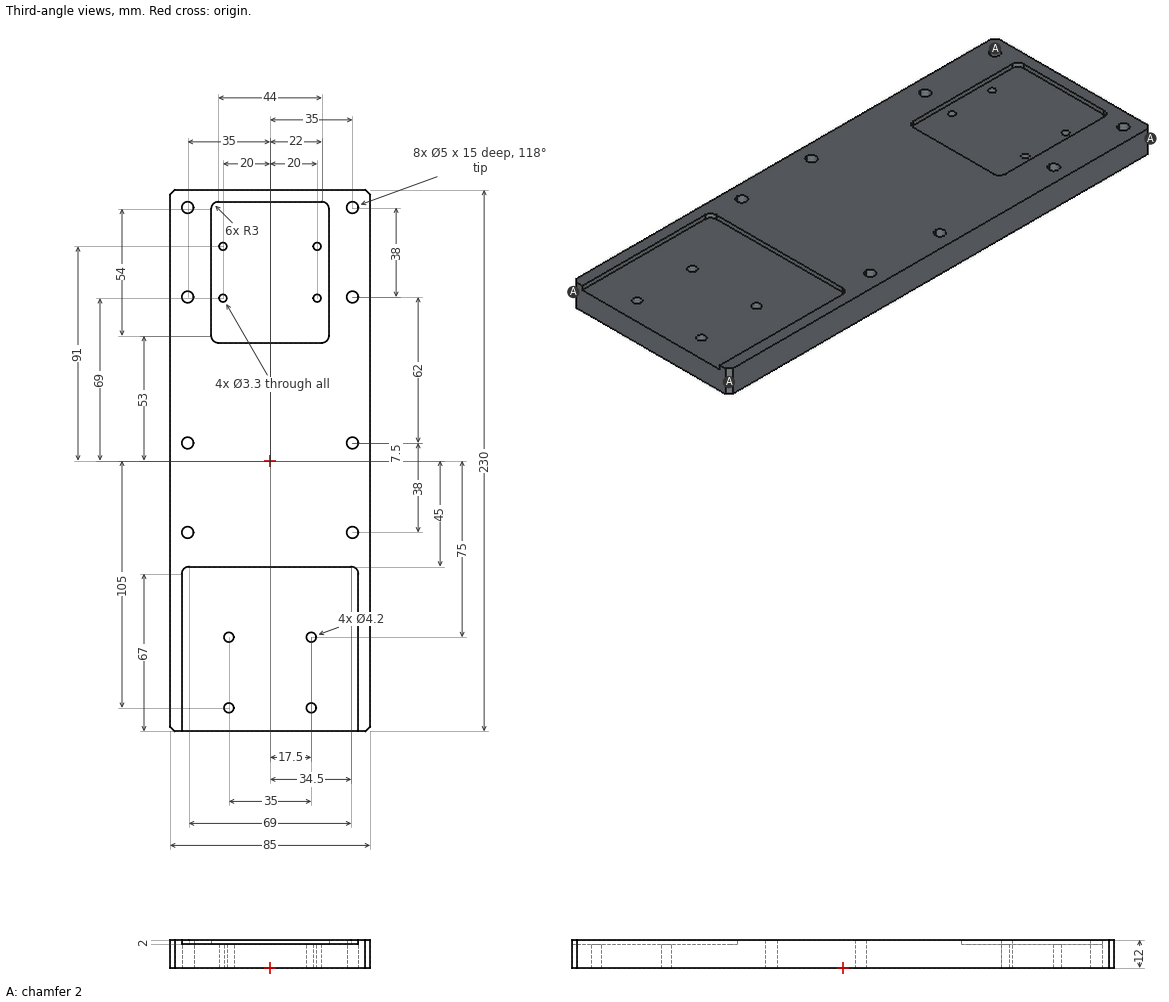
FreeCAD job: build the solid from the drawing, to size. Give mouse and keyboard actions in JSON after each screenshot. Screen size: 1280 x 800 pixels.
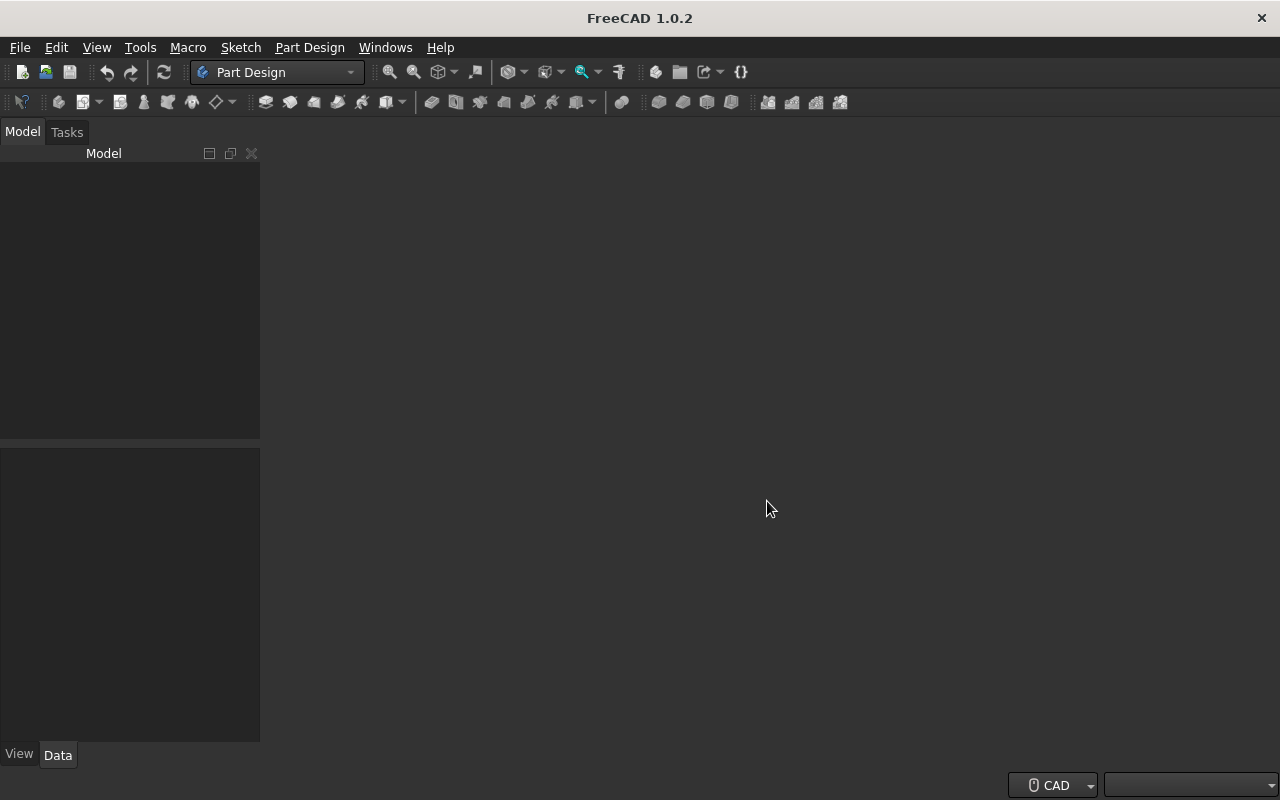
{"action": "key", "text": "ctrl+n"}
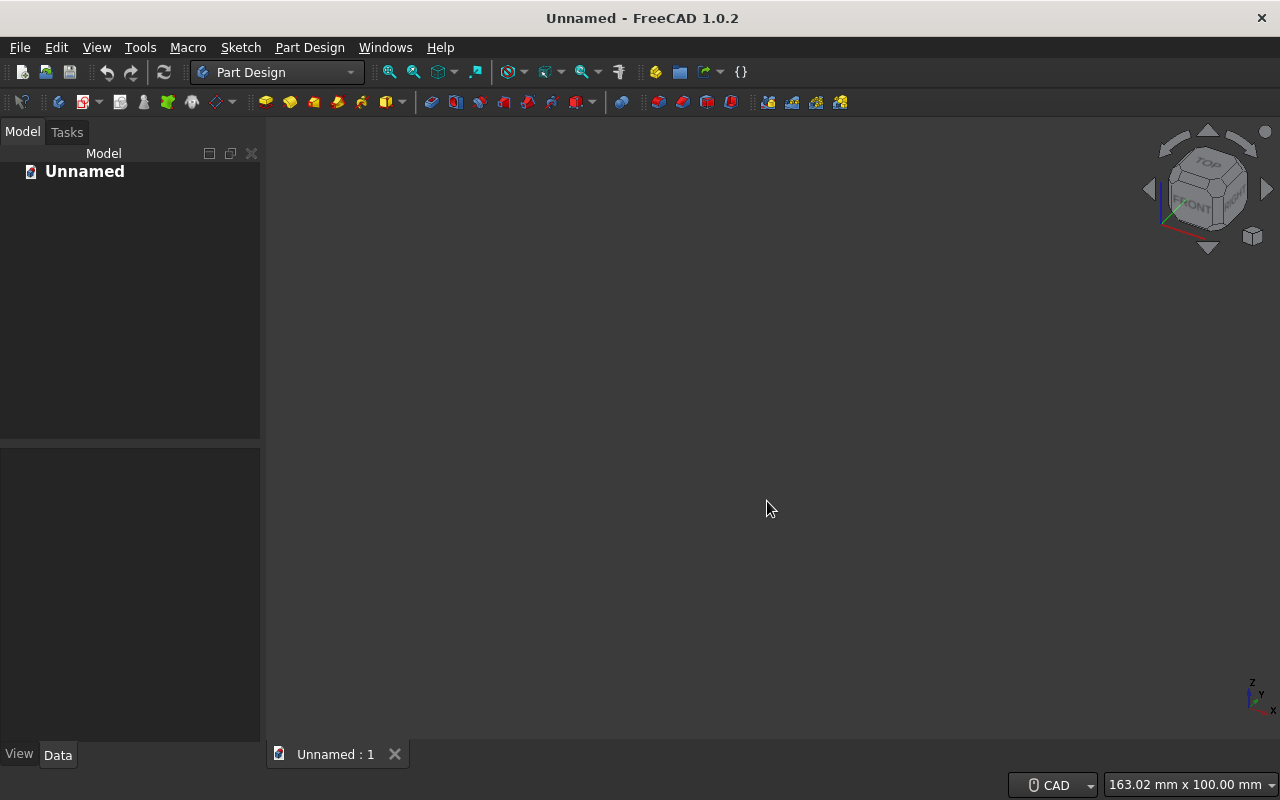
{"action": "left_click", "coordinate": [84, 102]}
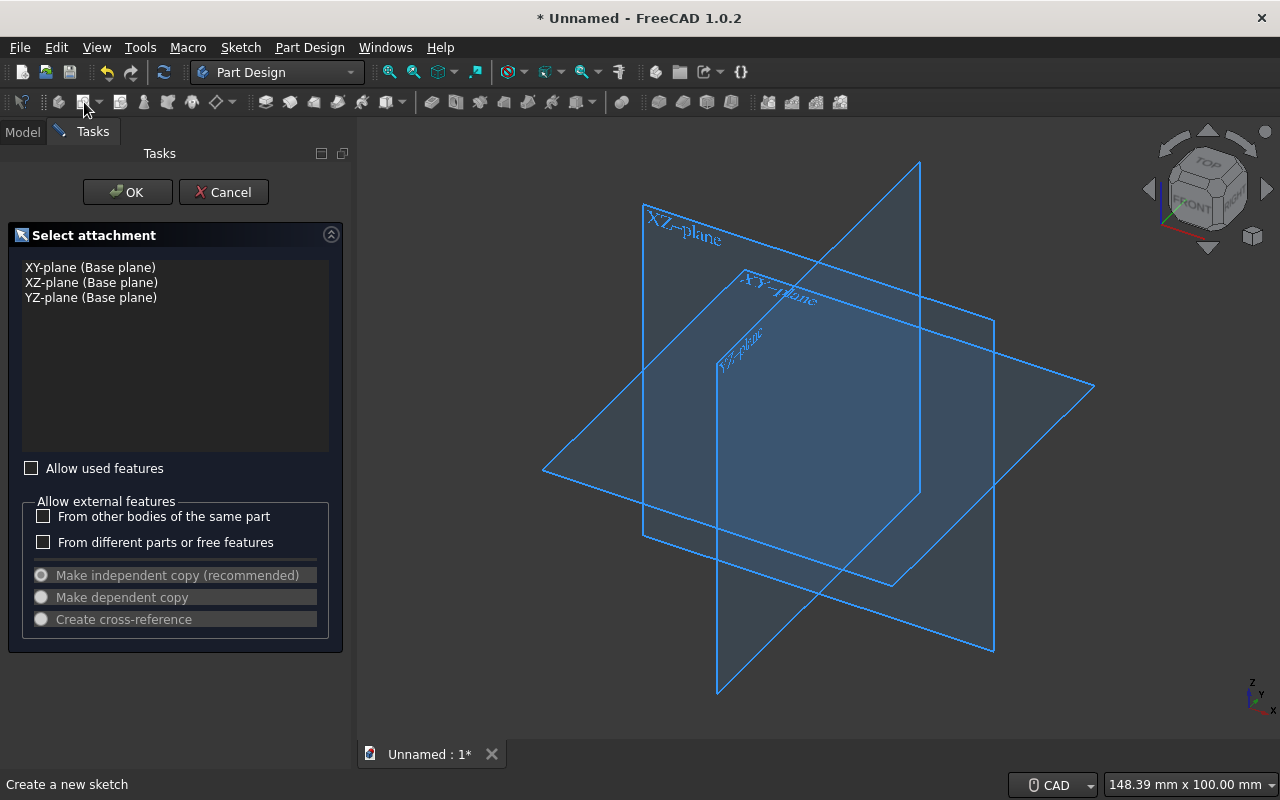
{"action": "left_click", "coordinate": [82, 268]}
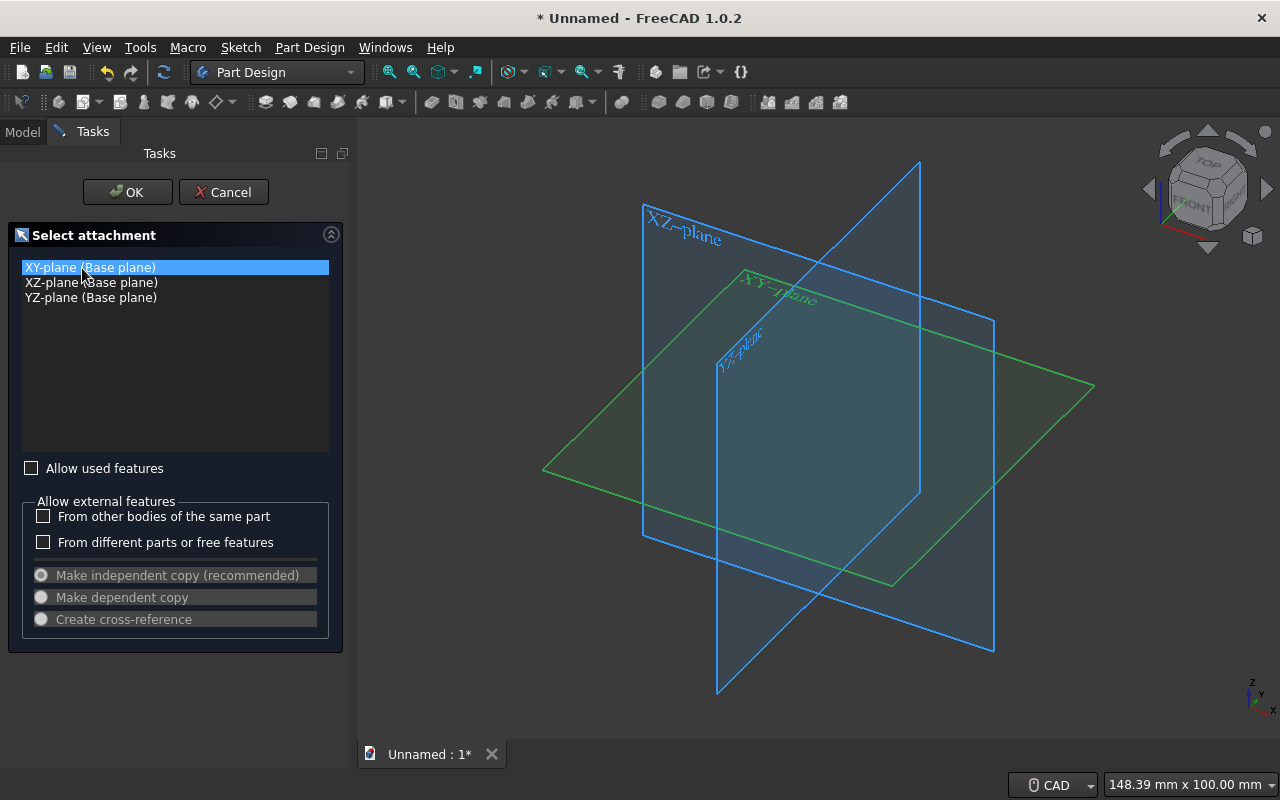
{"action": "left_click", "coordinate": [128, 192]}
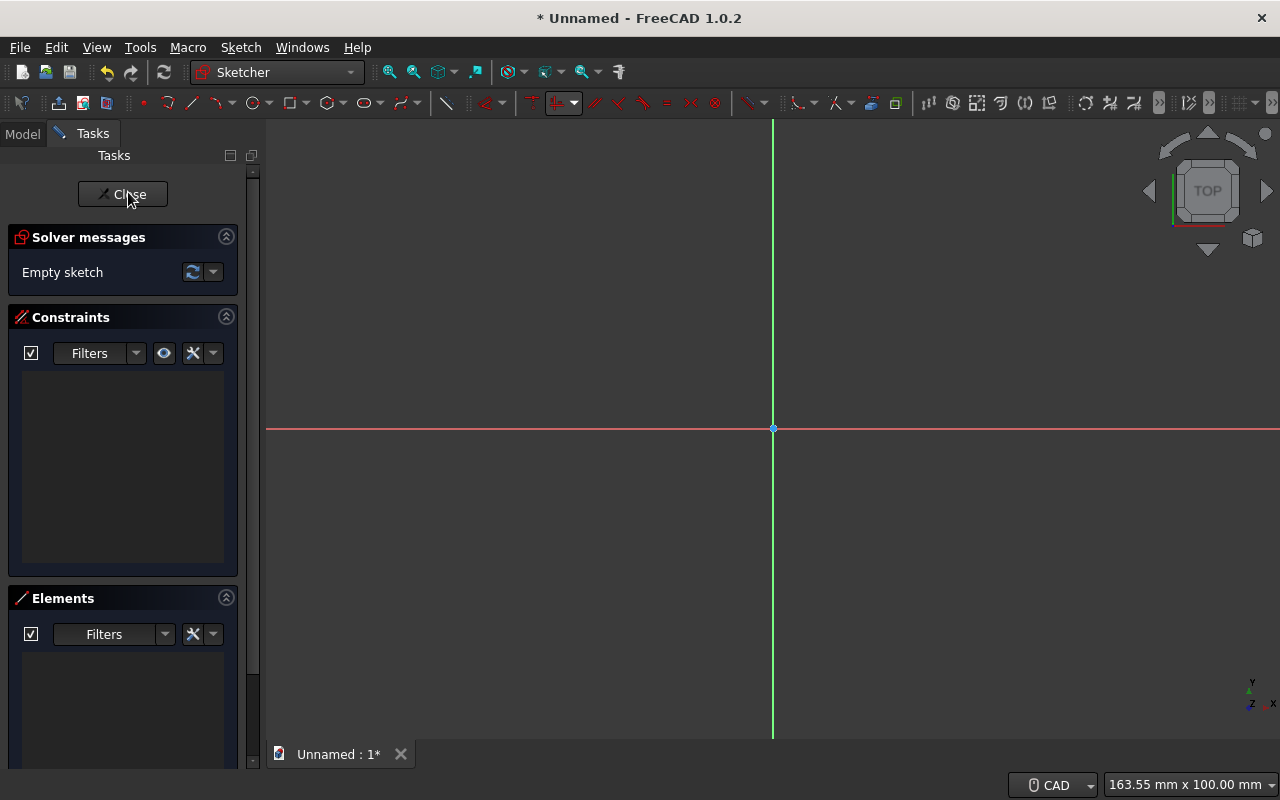
{"action": "scroll", "coordinate": [675, 429], "scroll_direction": "down", "scroll_amount": 6}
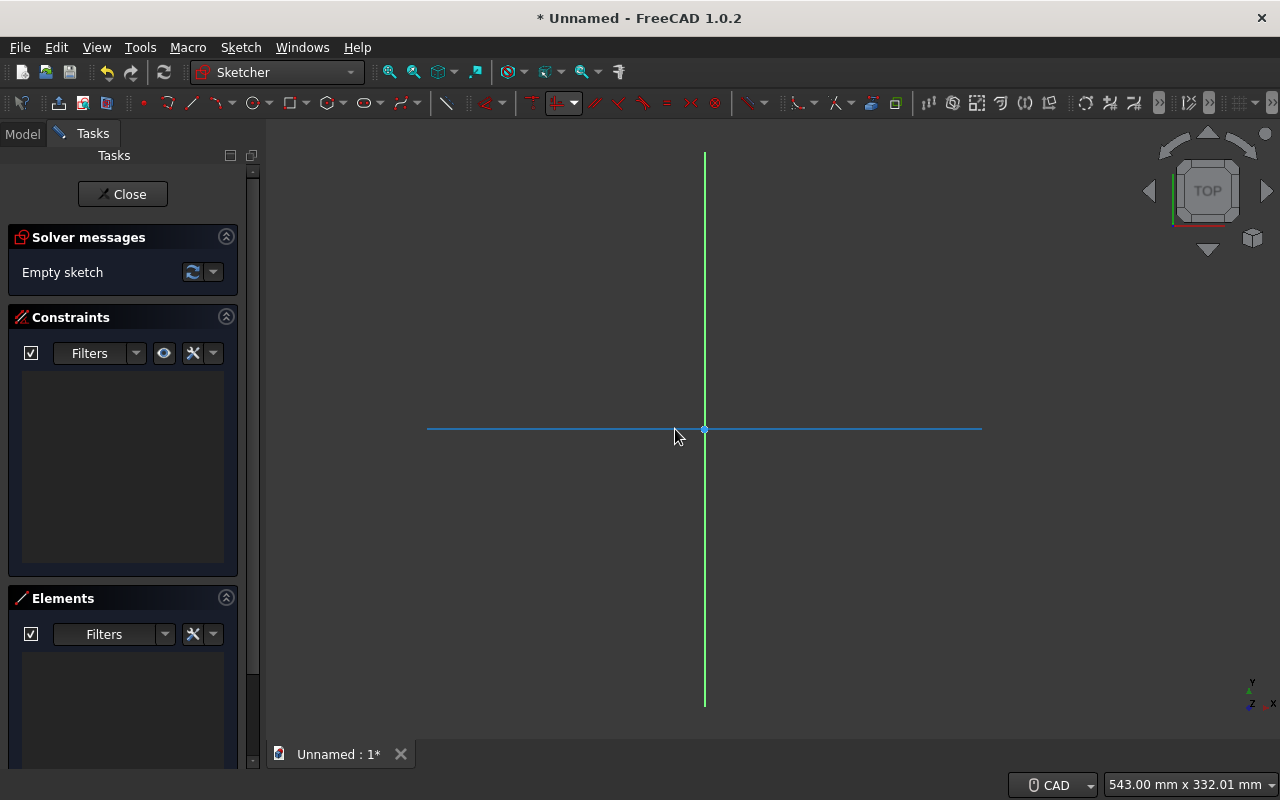
{"action": "key", "text": "g v"}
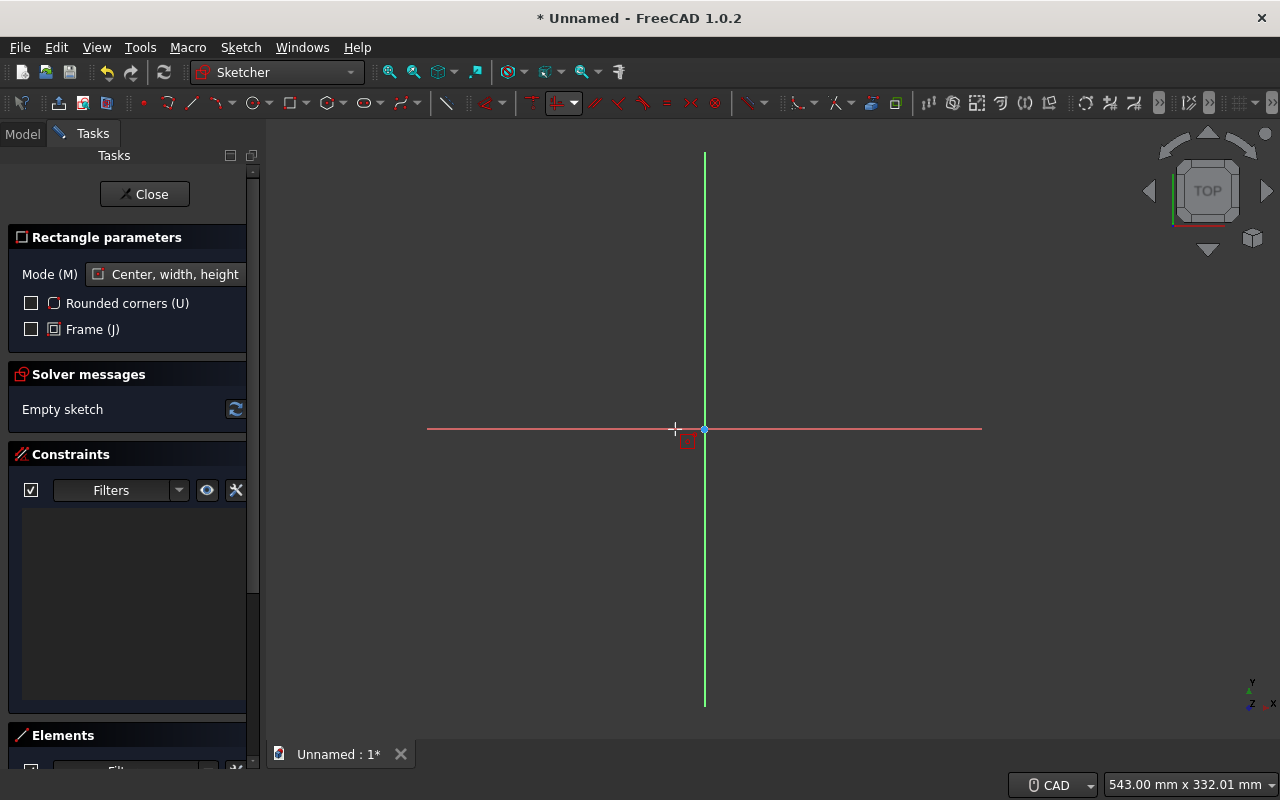
{"action": "left_click", "coordinate": [705, 429]}
{"action": "left_click", "coordinate": [784, 215]}
{"action": "key", "text": "Escape"}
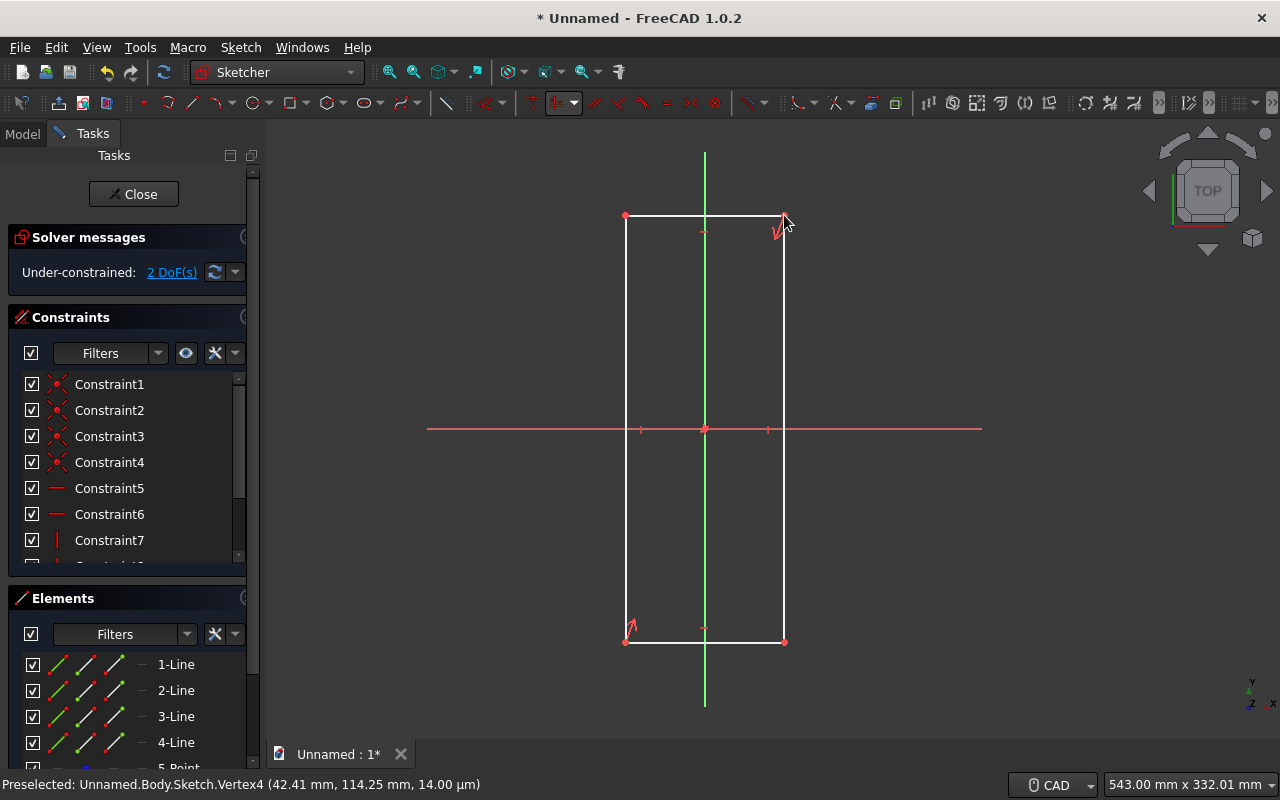
{"action": "left_click", "coordinate": [673, 643]}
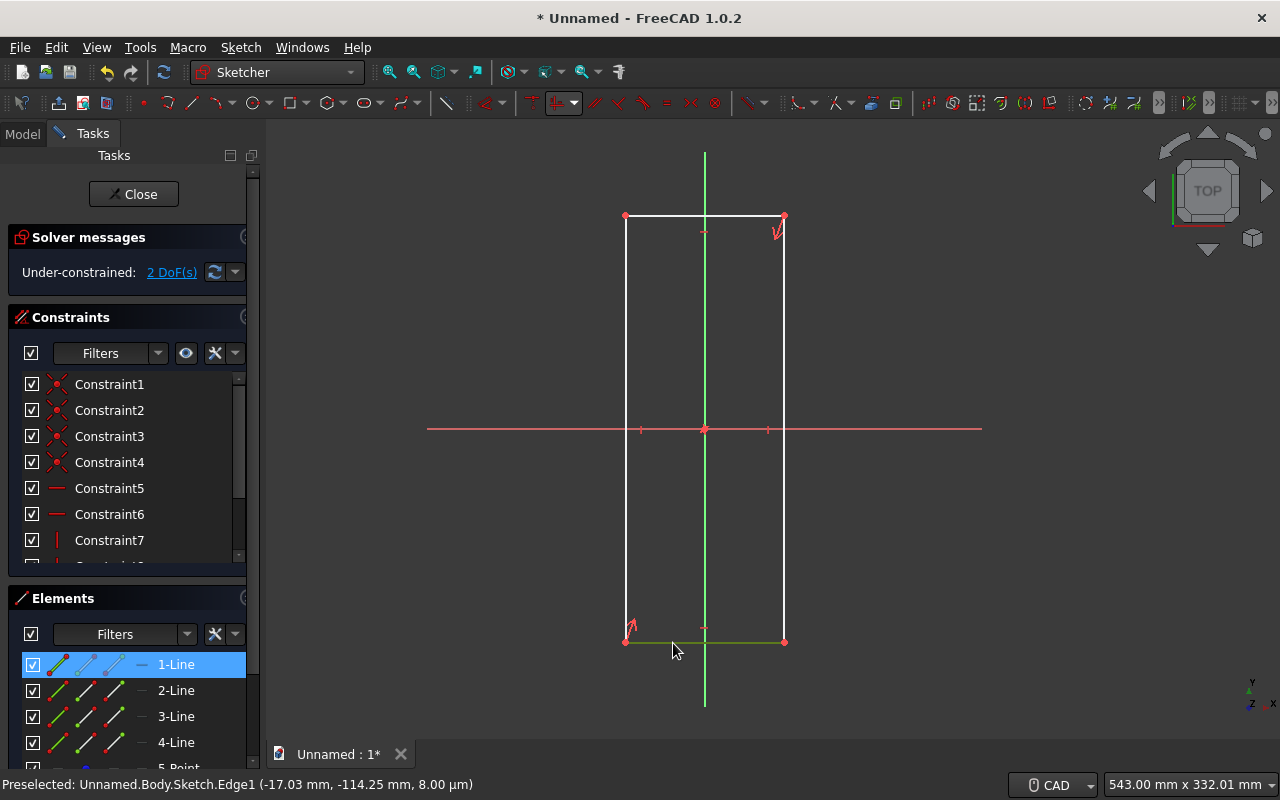
{"action": "key", "text": "l"}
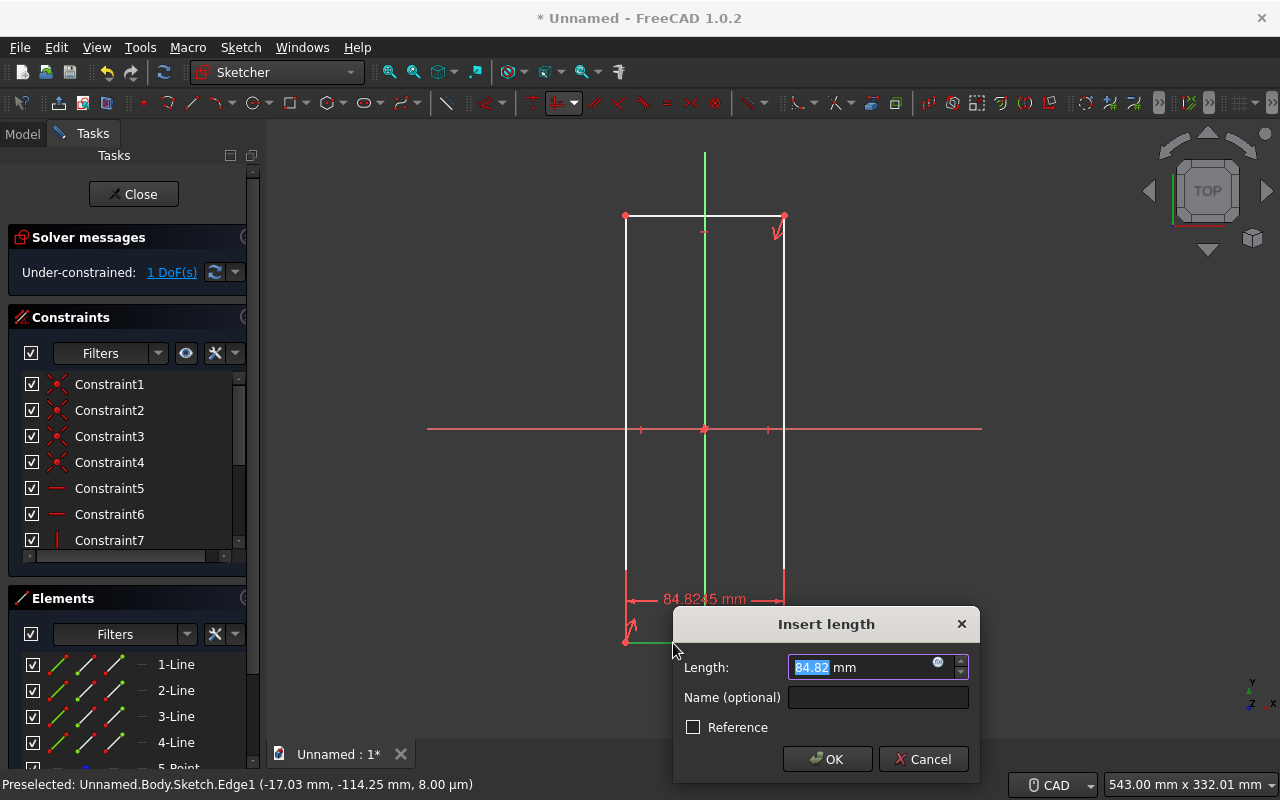
{"action": "type", "text": "85"}
{"action": "key", "text": "Return"}